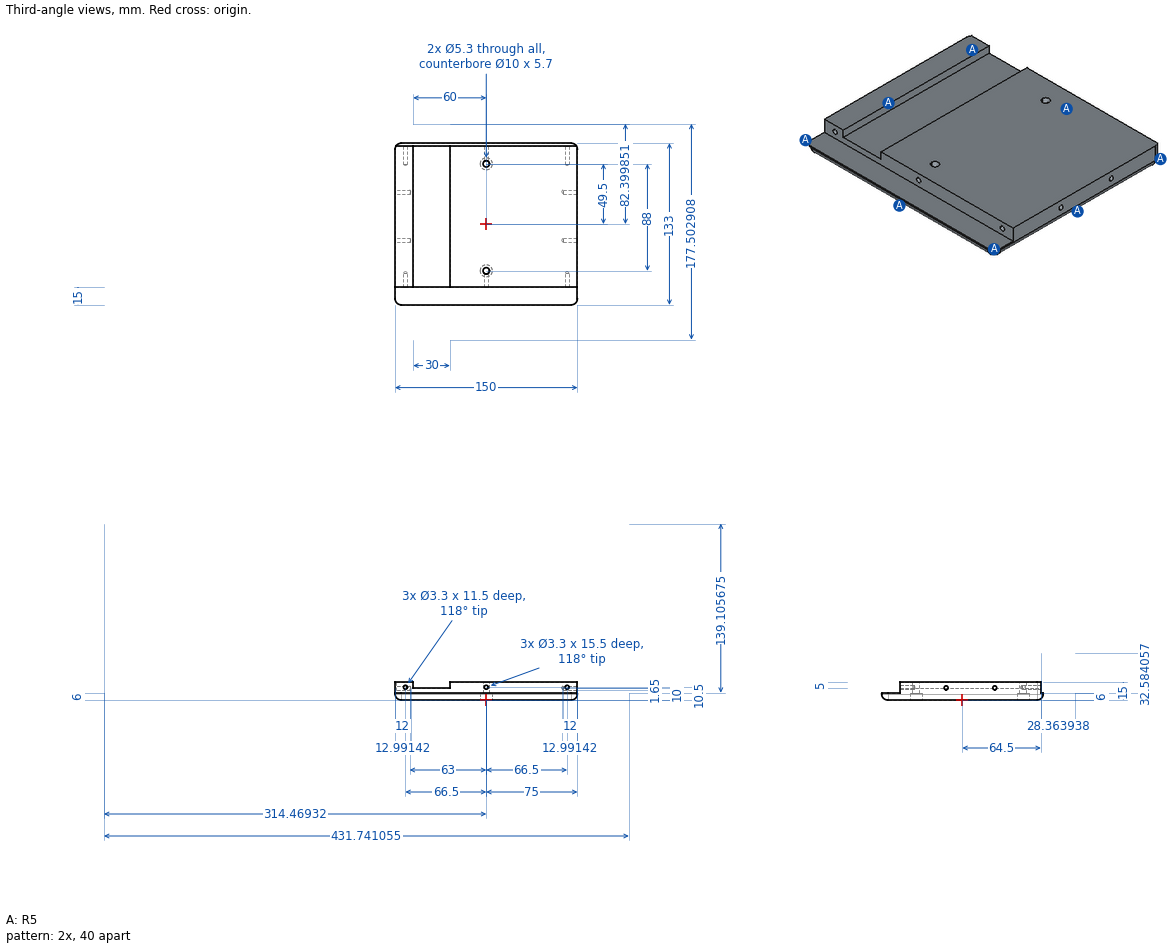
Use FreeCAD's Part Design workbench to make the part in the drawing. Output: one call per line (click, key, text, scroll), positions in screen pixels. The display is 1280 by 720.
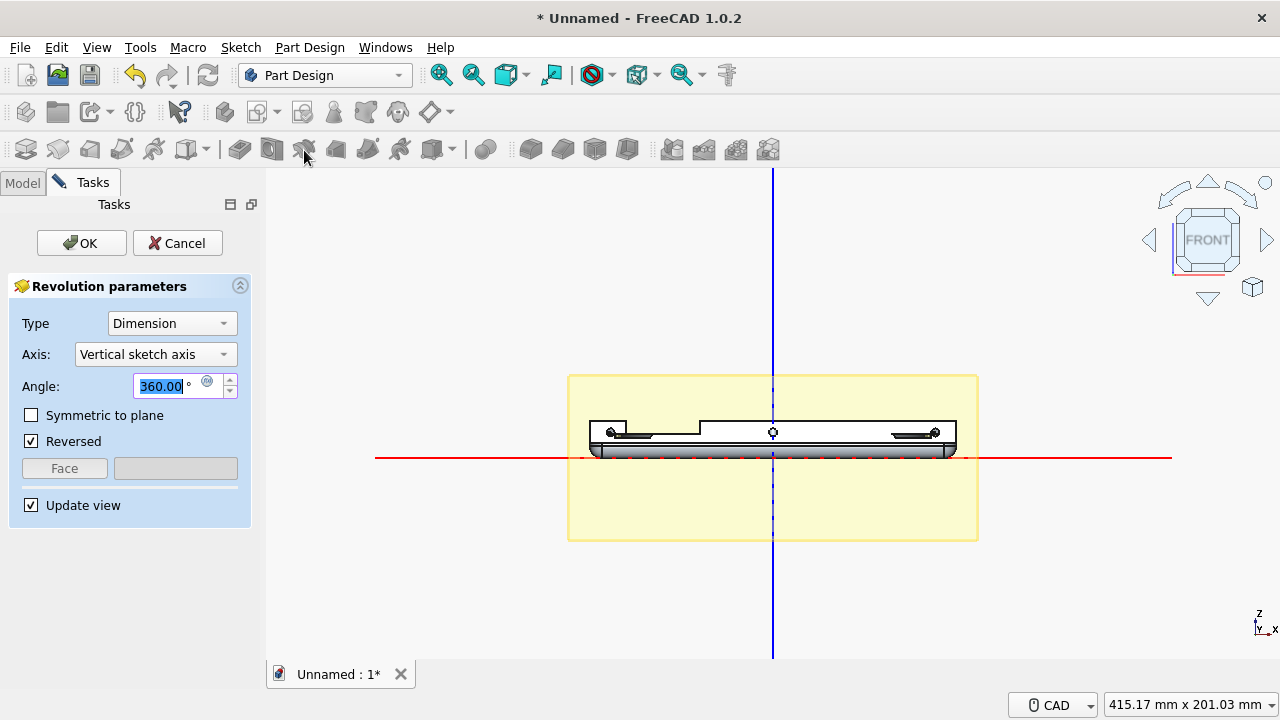
click(156, 354)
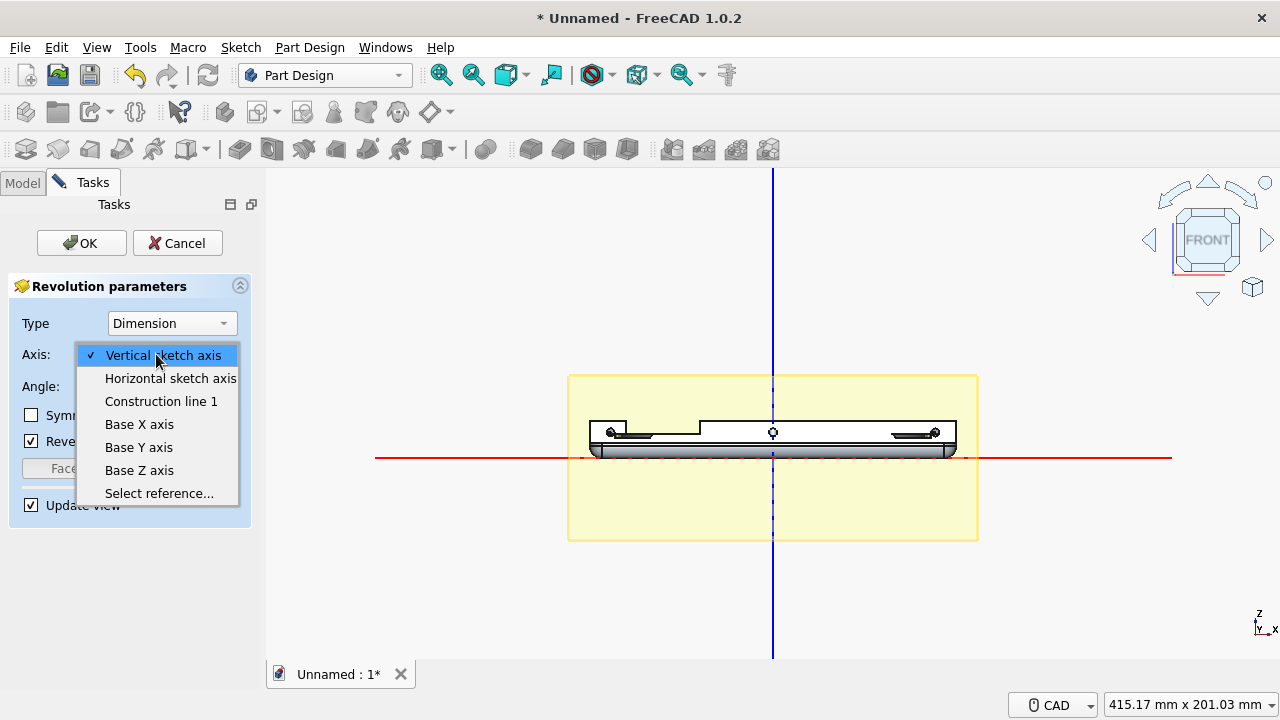
click(156, 402)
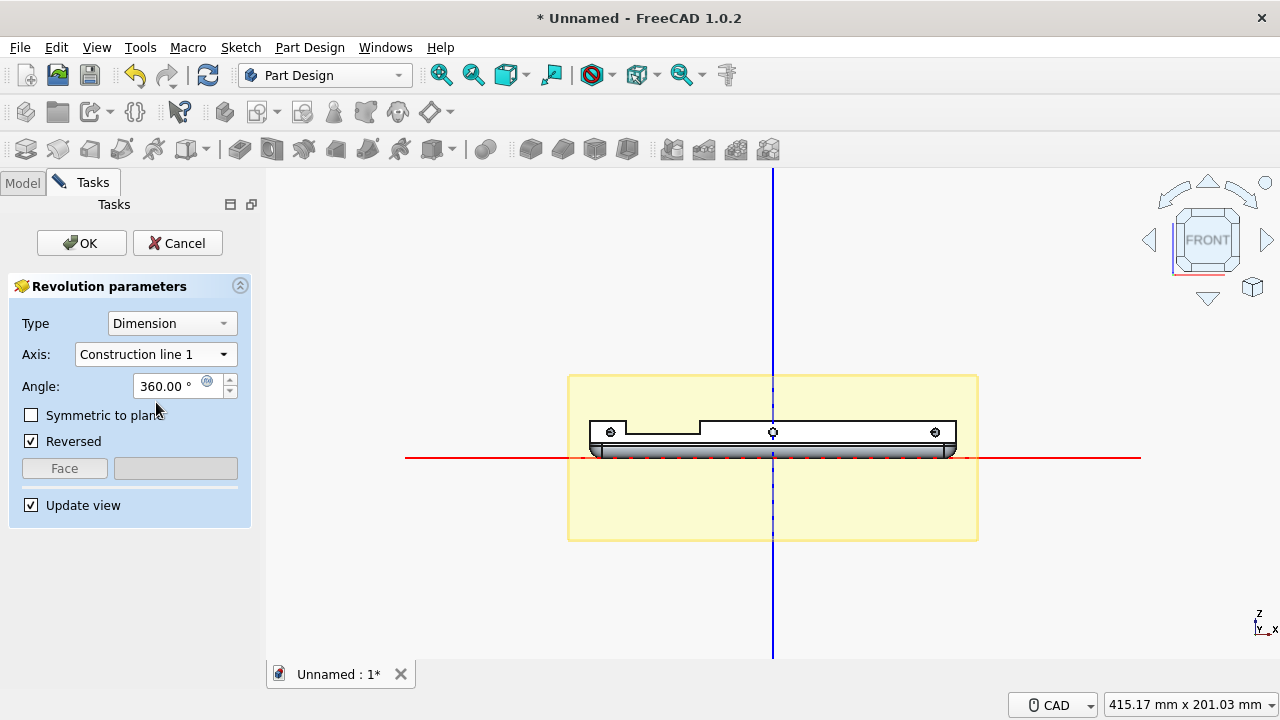
click(82, 243)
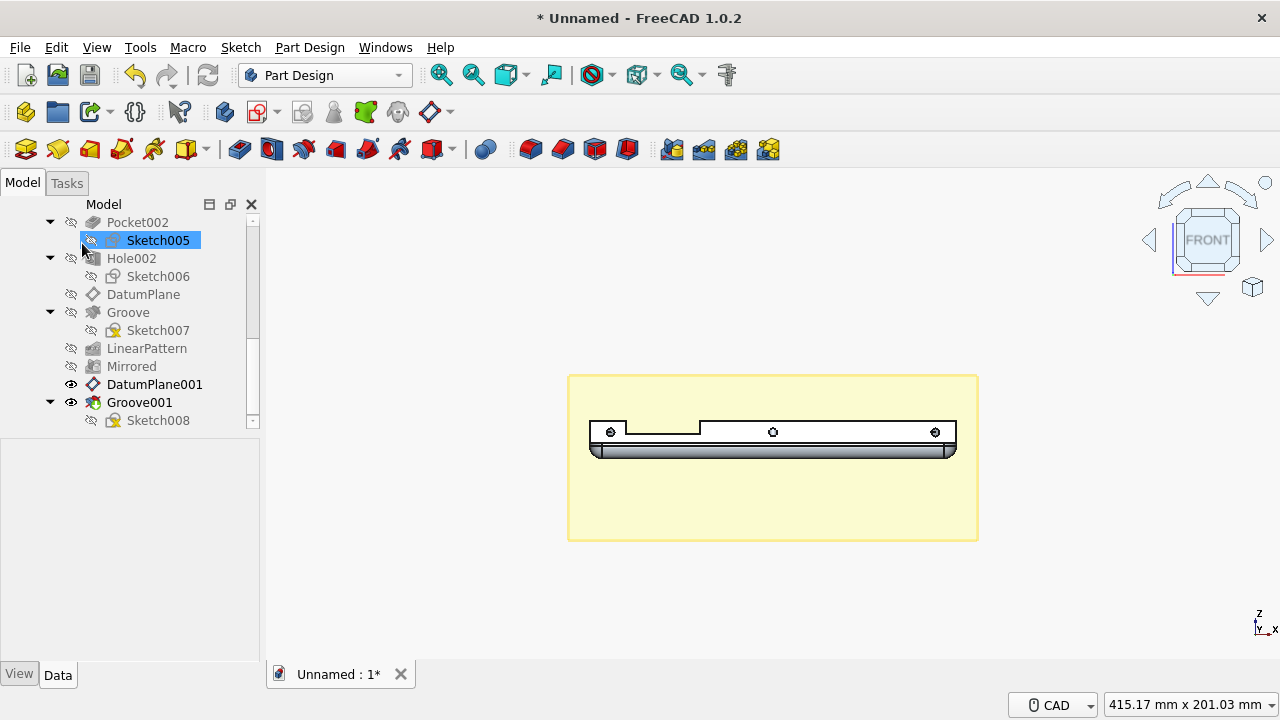
click(116, 384)
key(space)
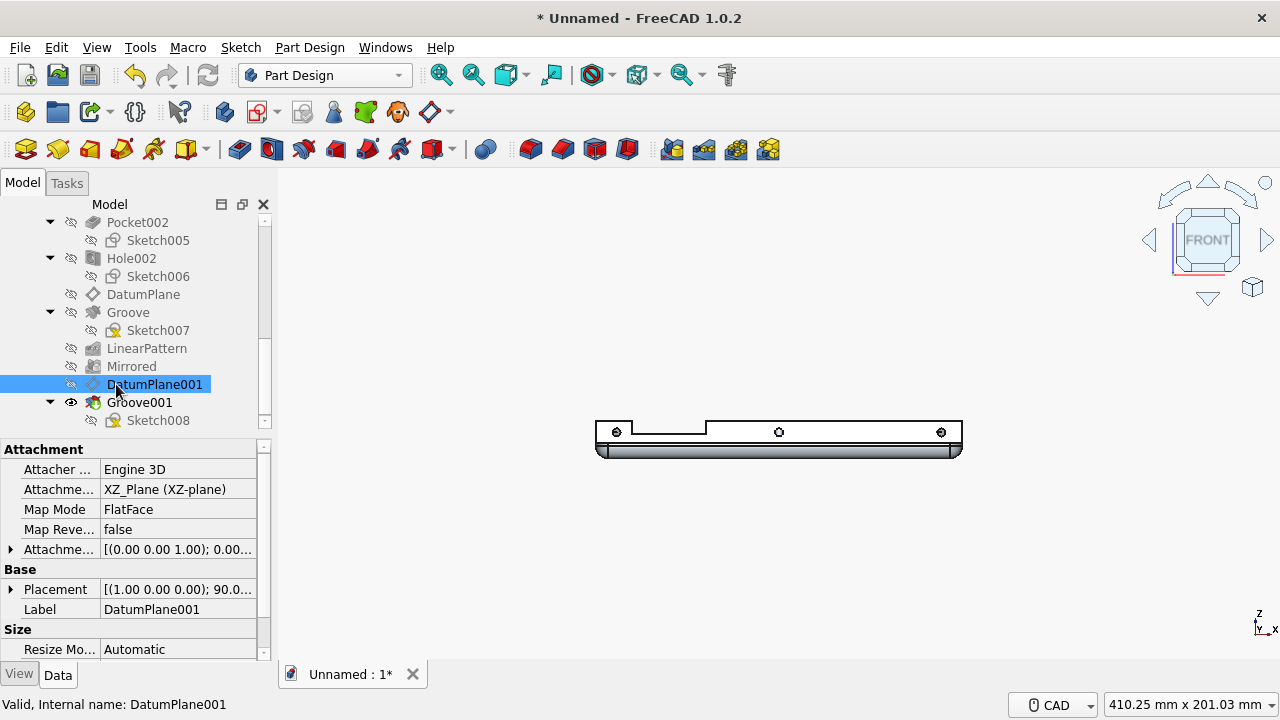
key(0)